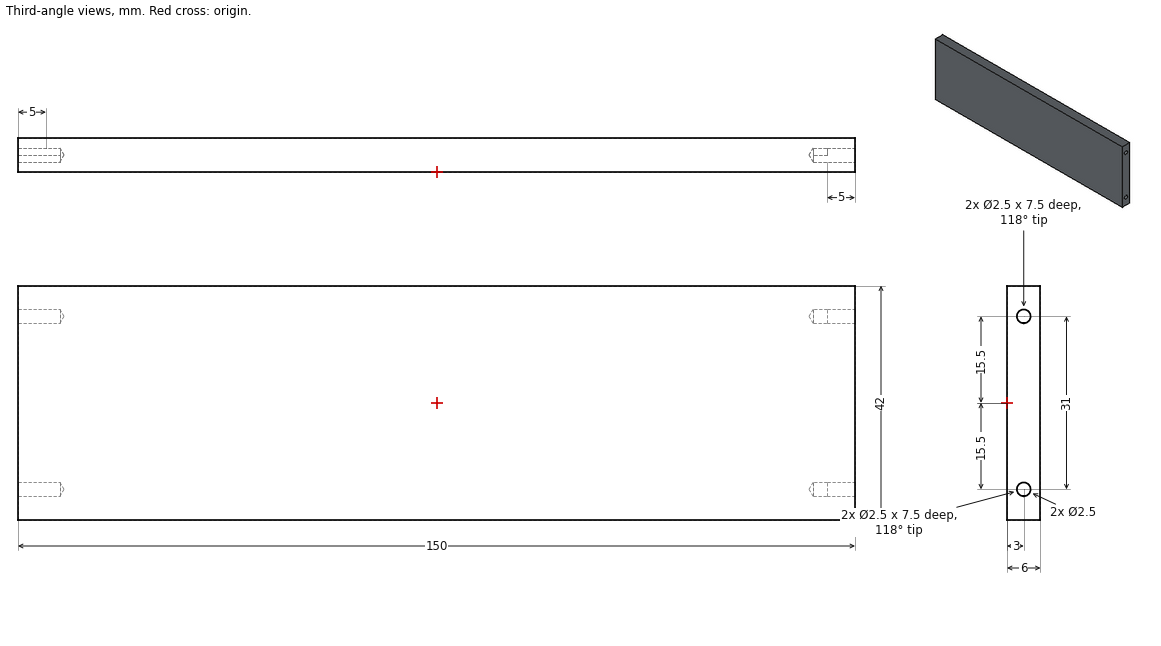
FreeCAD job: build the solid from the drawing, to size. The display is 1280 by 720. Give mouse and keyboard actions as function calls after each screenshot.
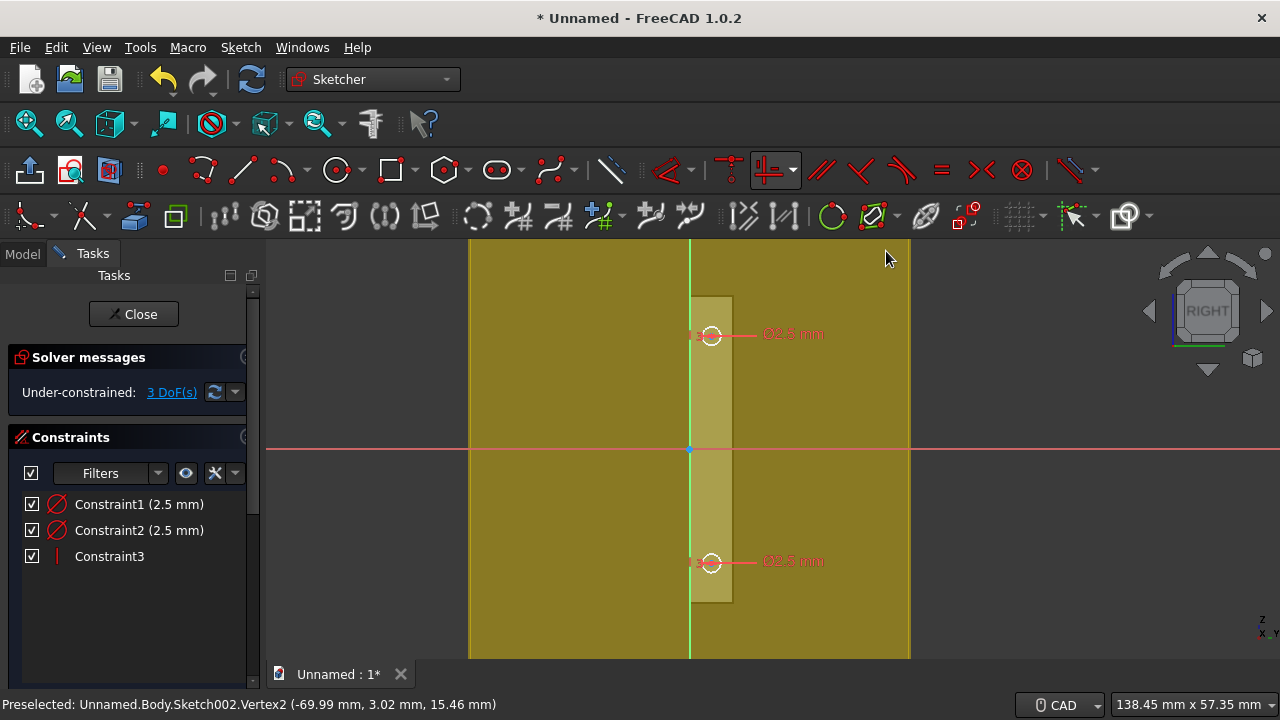
click(666, 170)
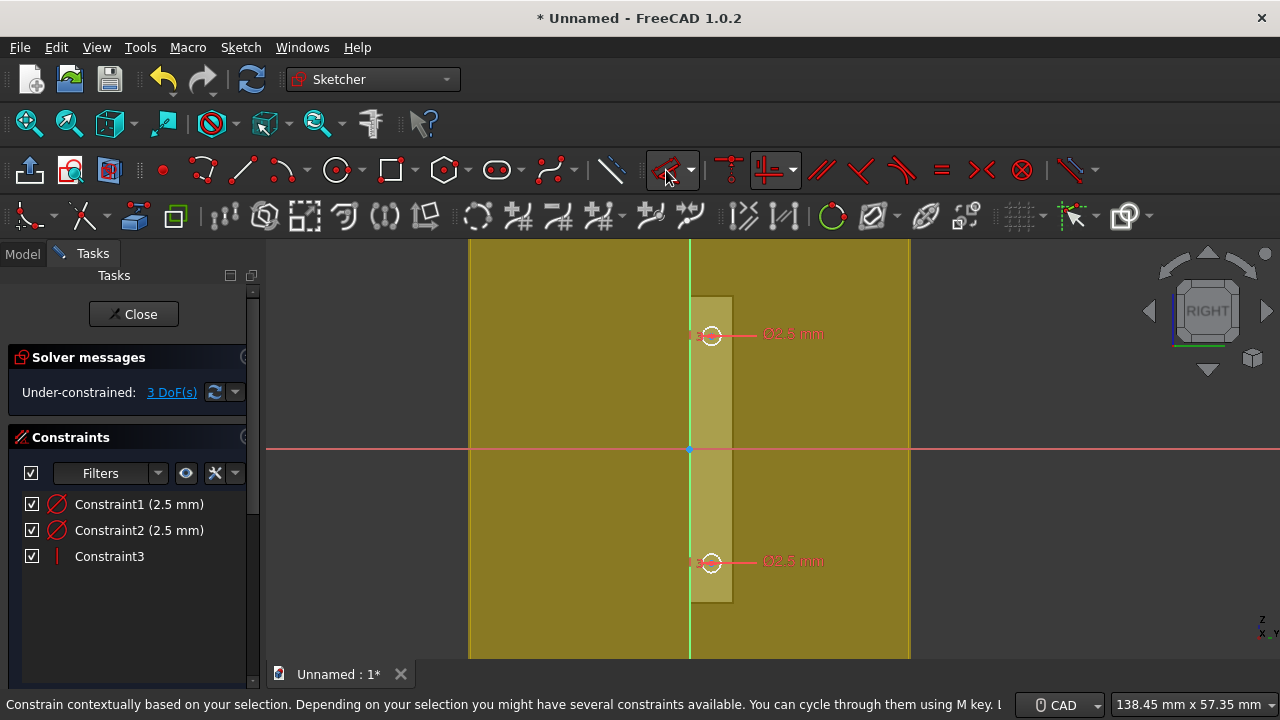
scroll(712, 563, up, 3)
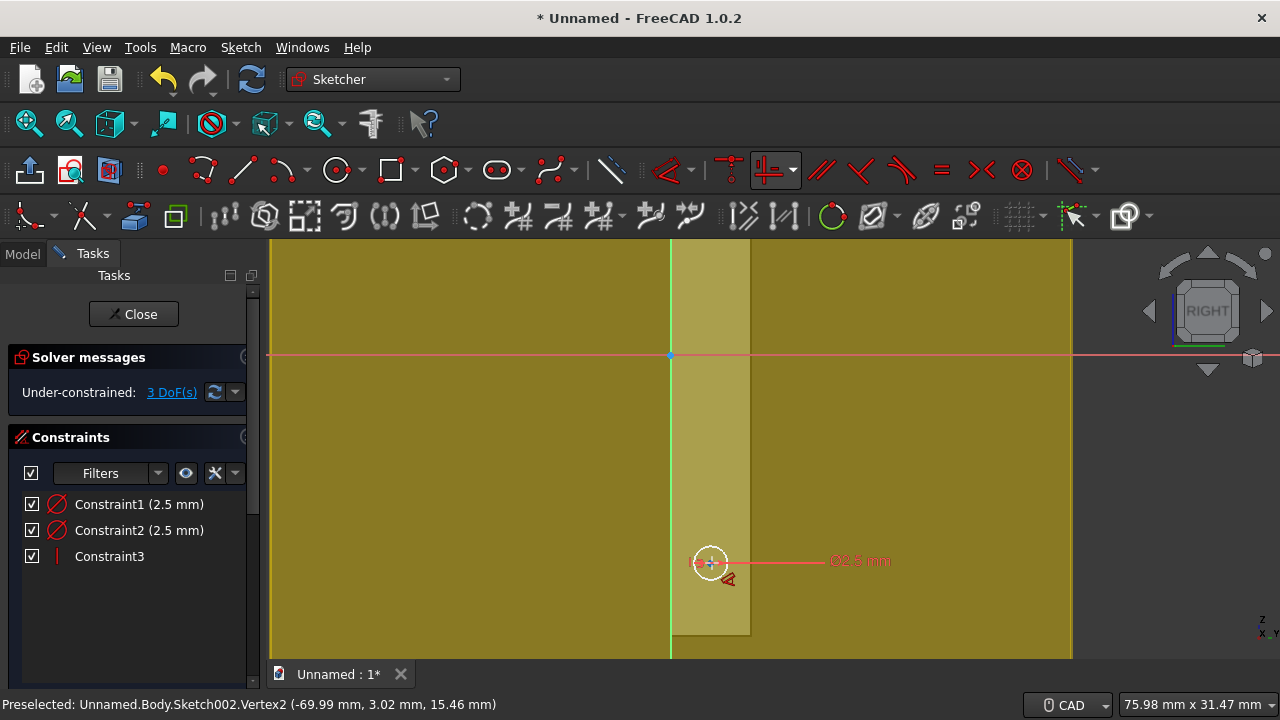
click(711, 563)
click(691, 597)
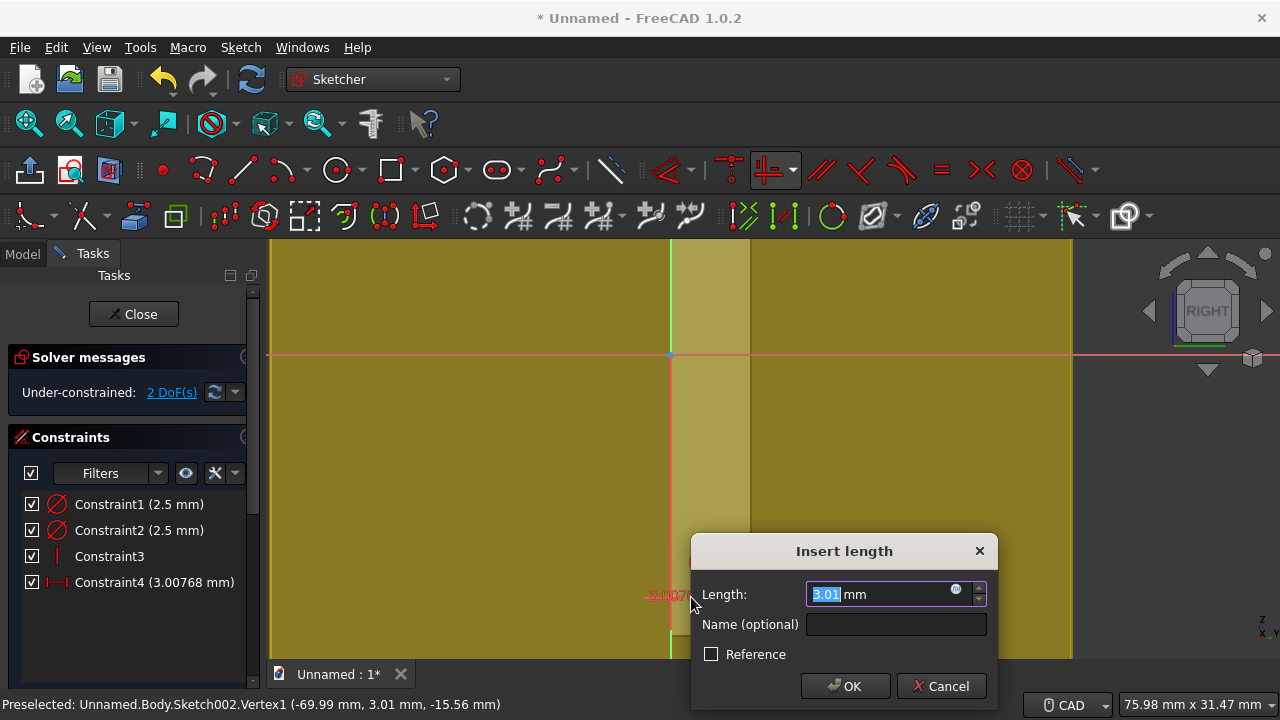
text(3)
key(Return)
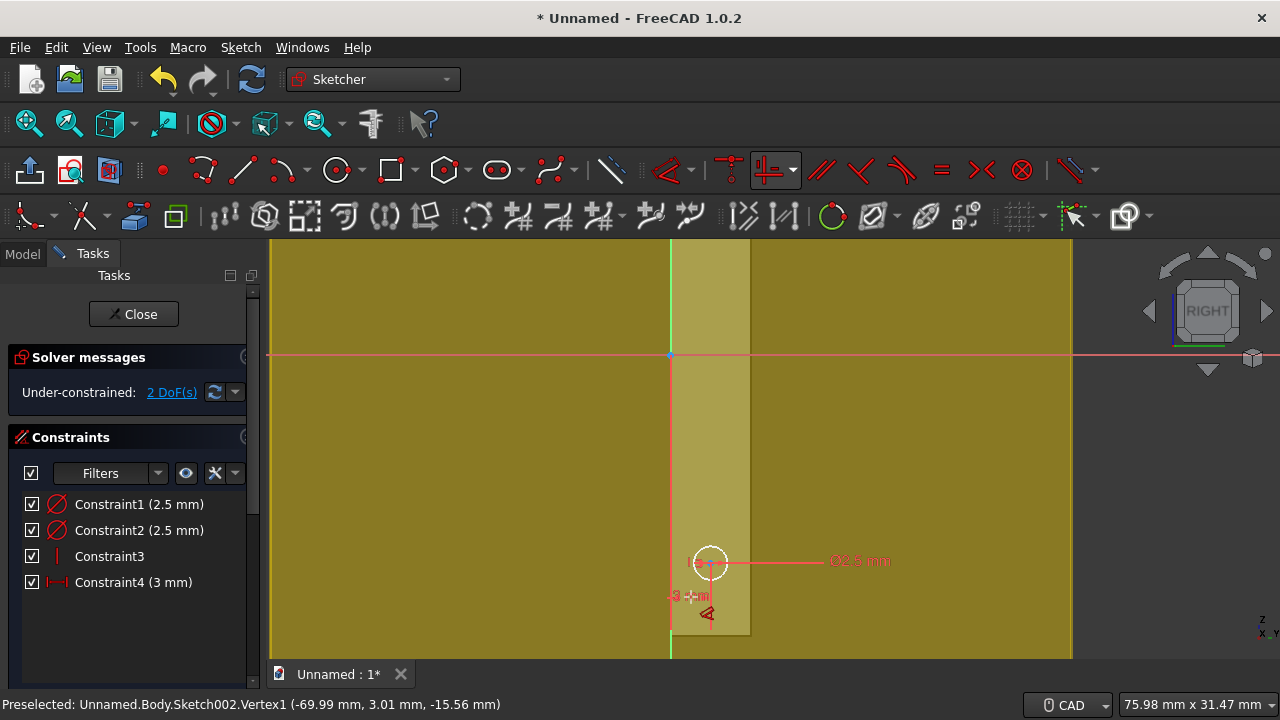
click(711, 563)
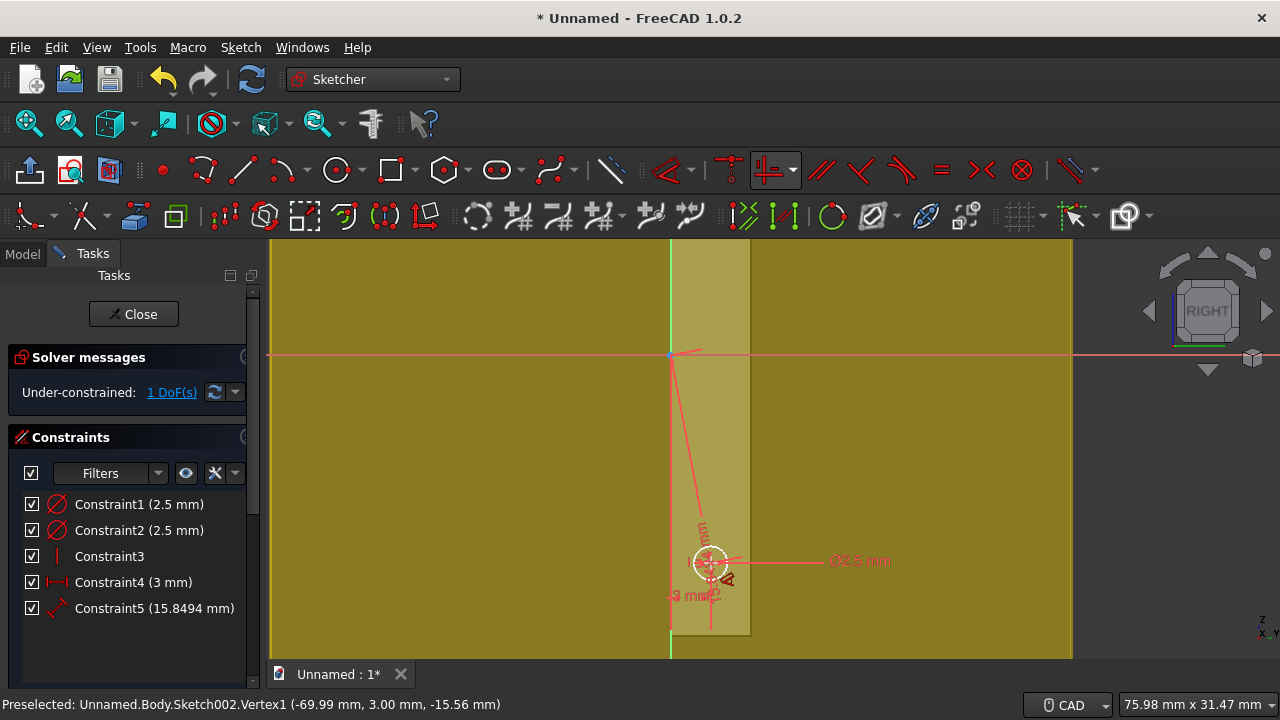
scroll(711, 563, down, 3)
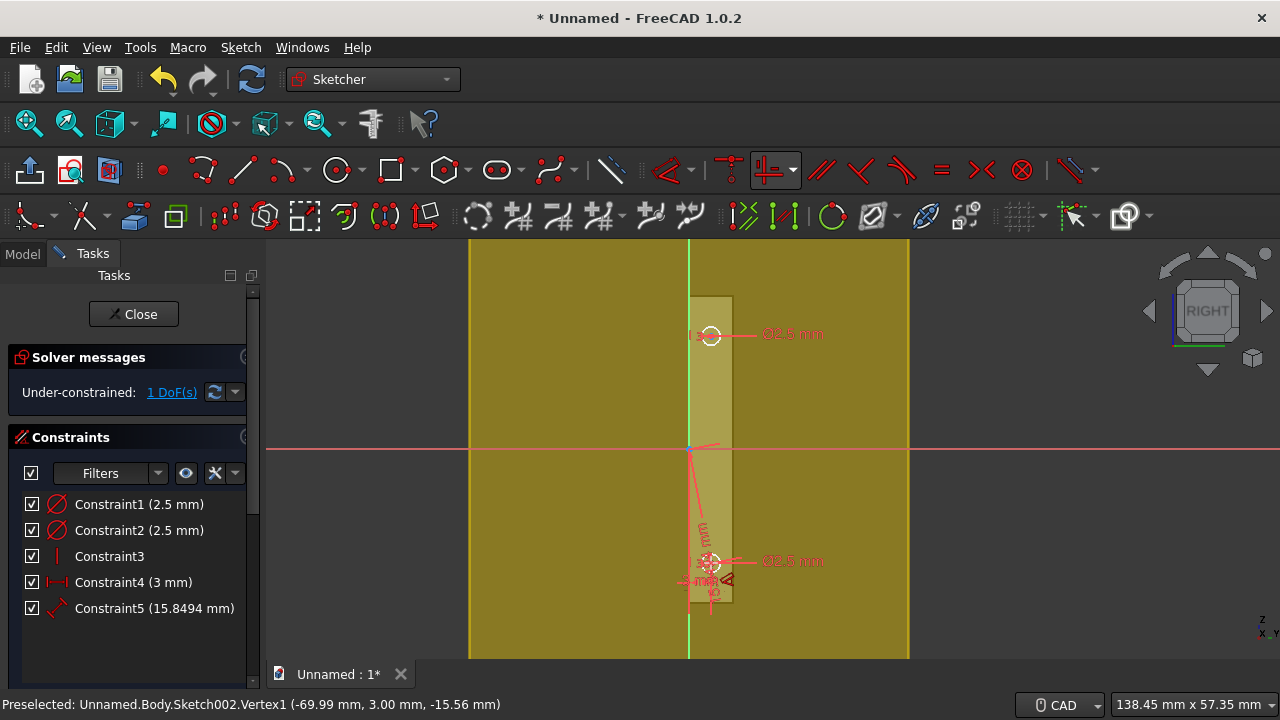
click(711, 336)
click(745, 398)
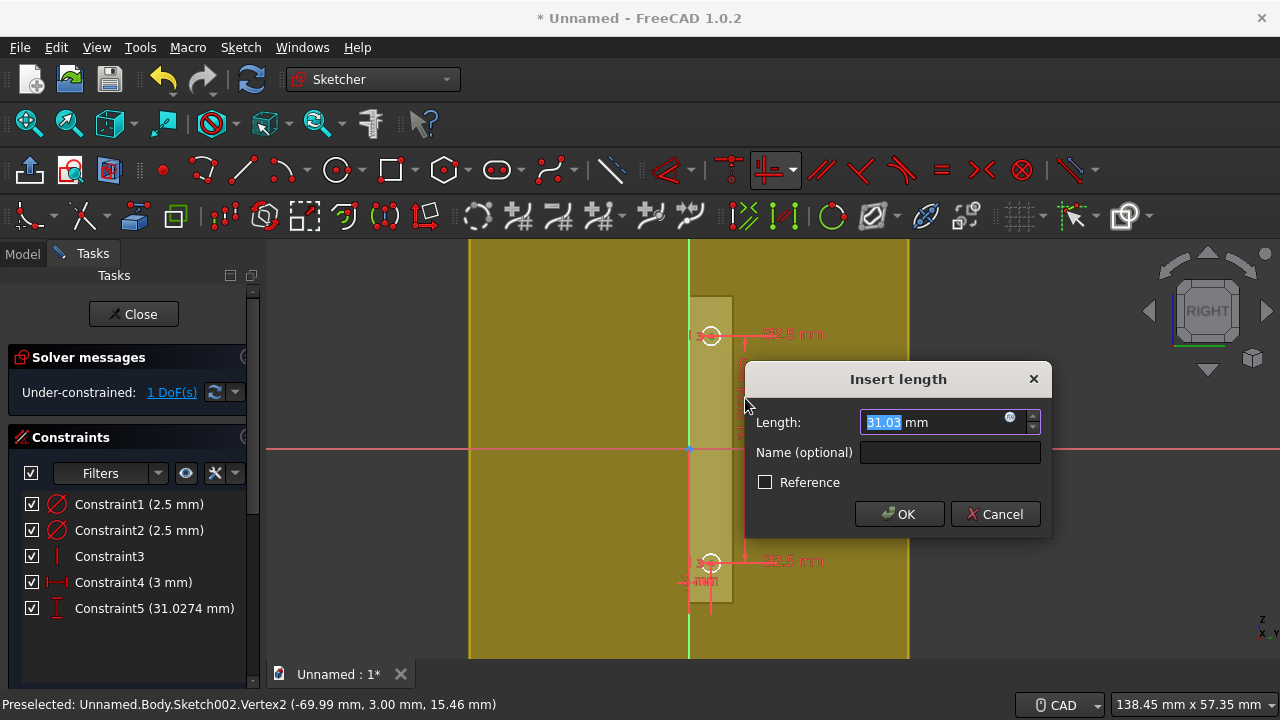
text(31)
key(Return)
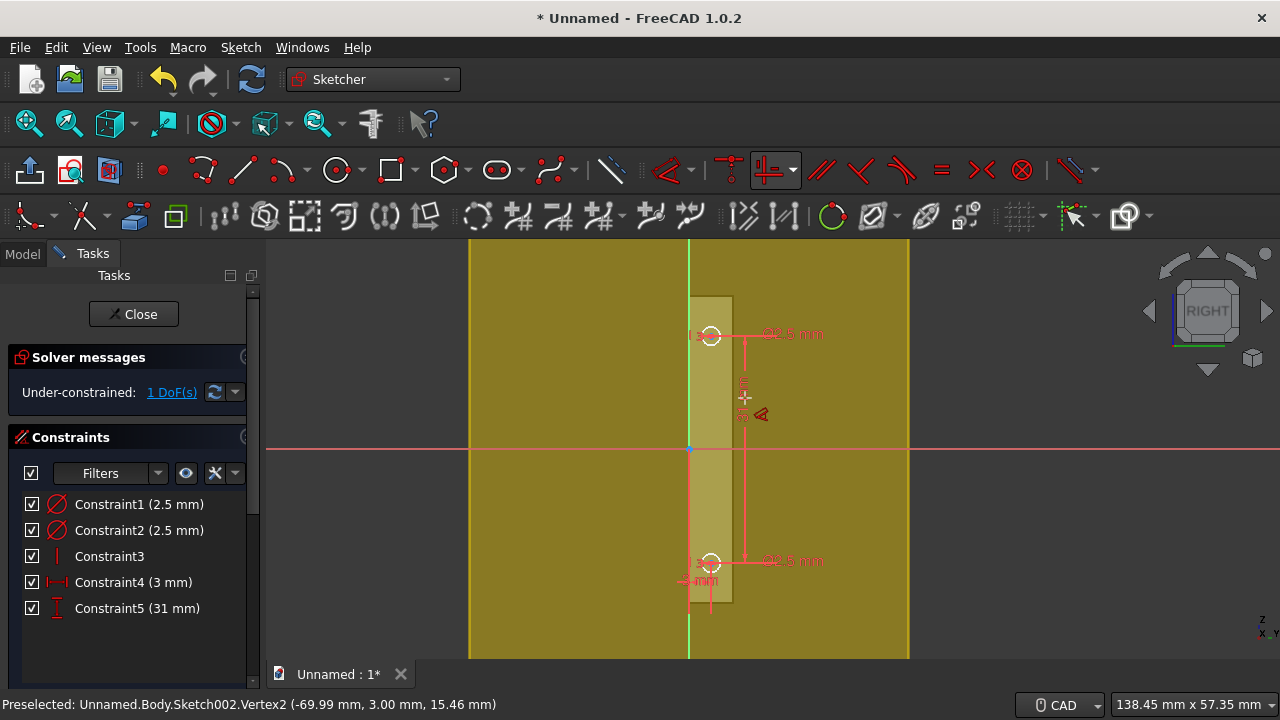
click(711, 563)
click(655, 506)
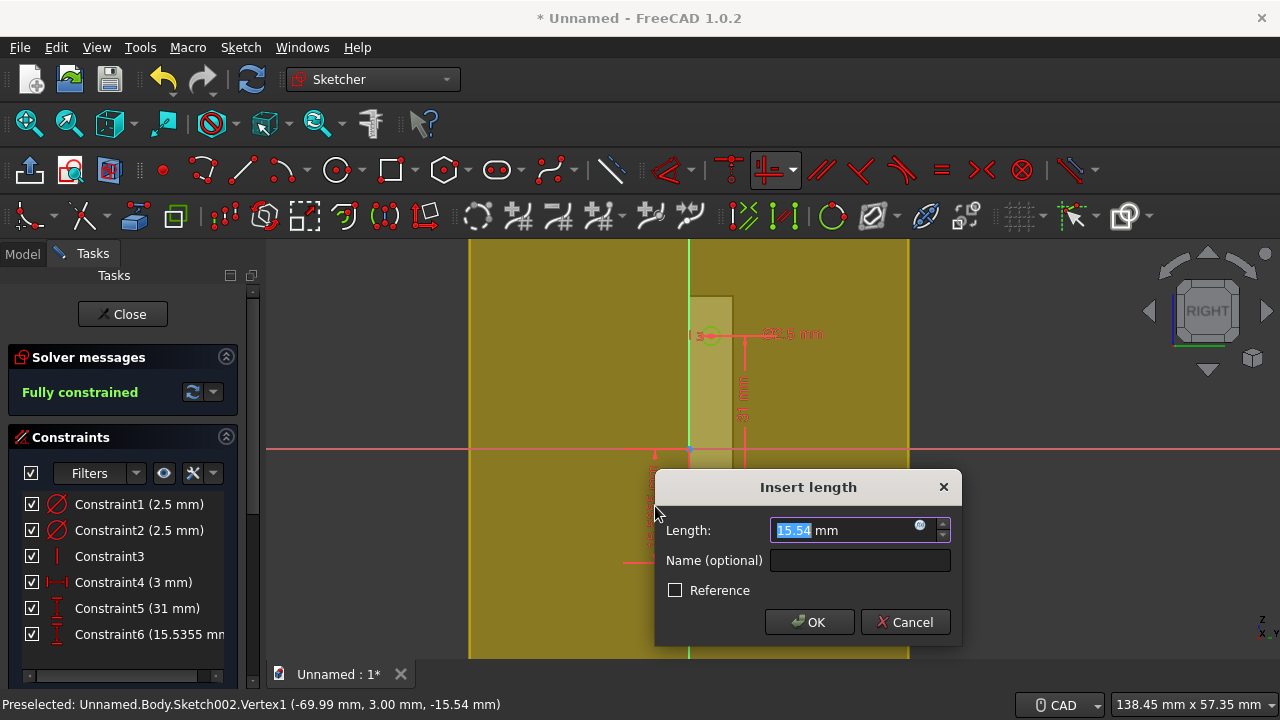
text(15.5)
key(Return)
key(Escape)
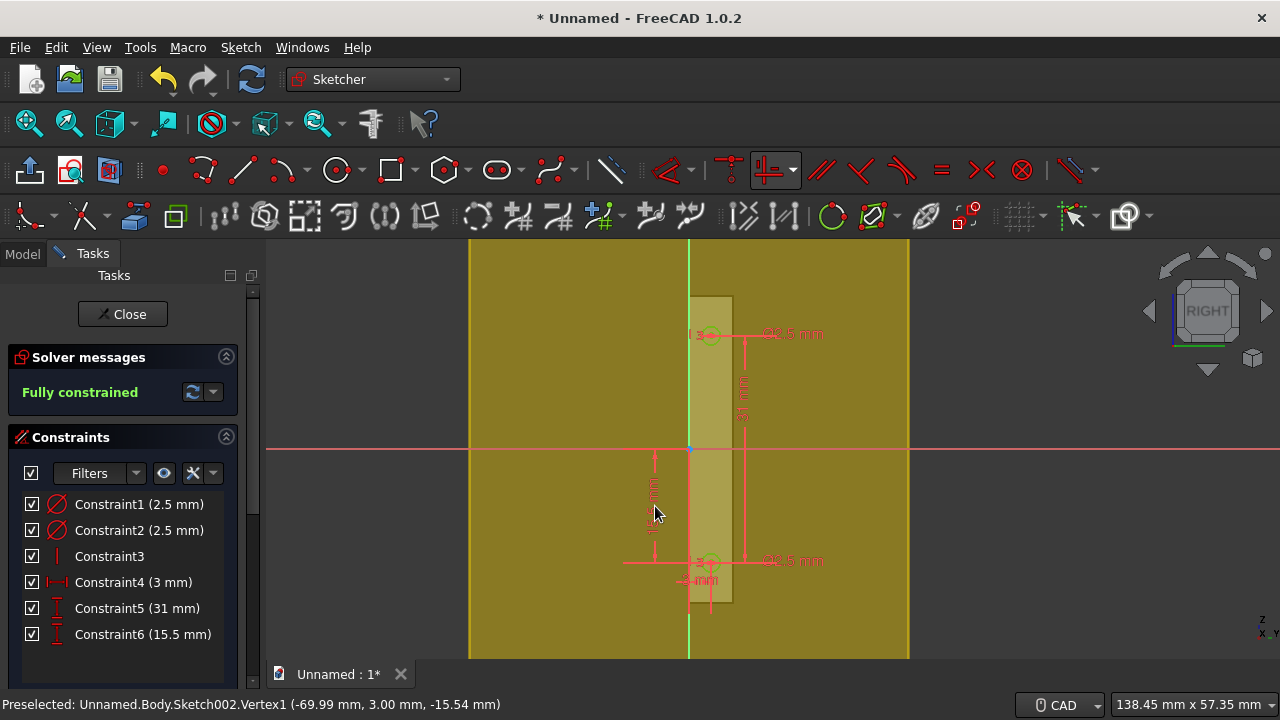
click(123, 314)